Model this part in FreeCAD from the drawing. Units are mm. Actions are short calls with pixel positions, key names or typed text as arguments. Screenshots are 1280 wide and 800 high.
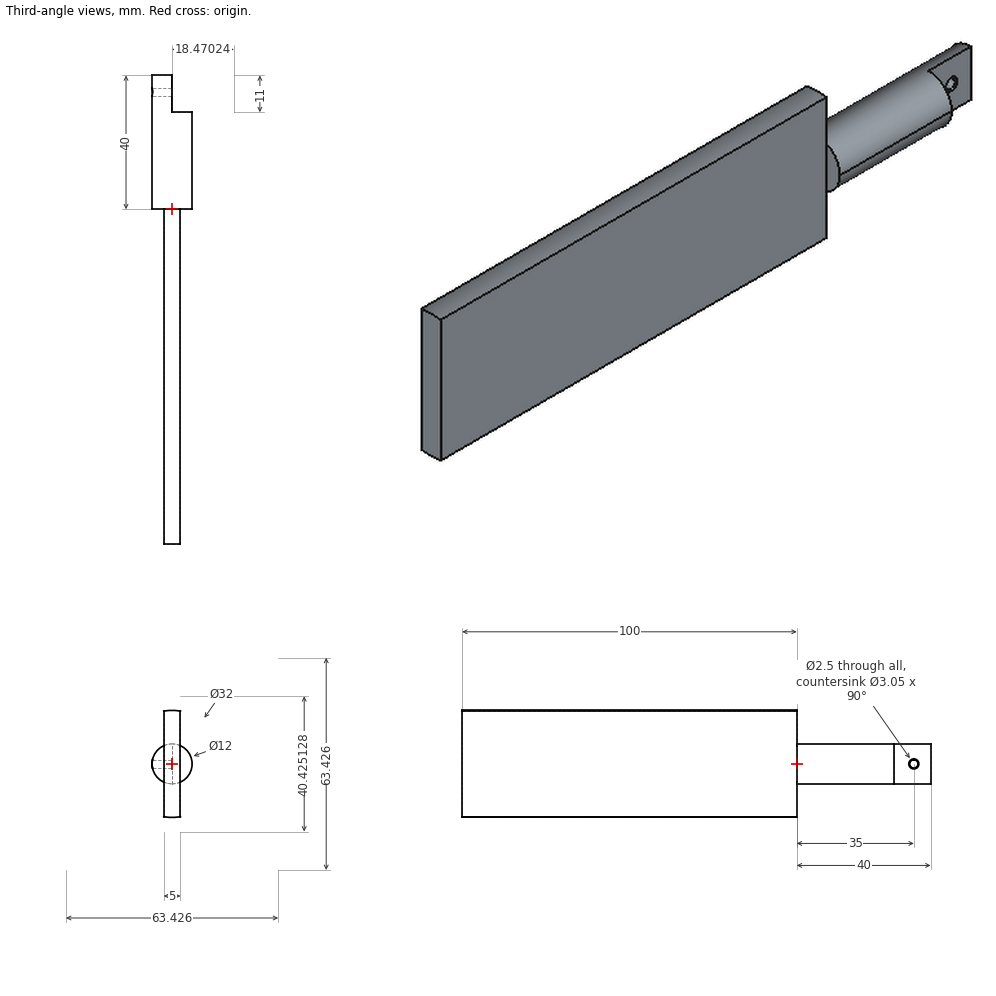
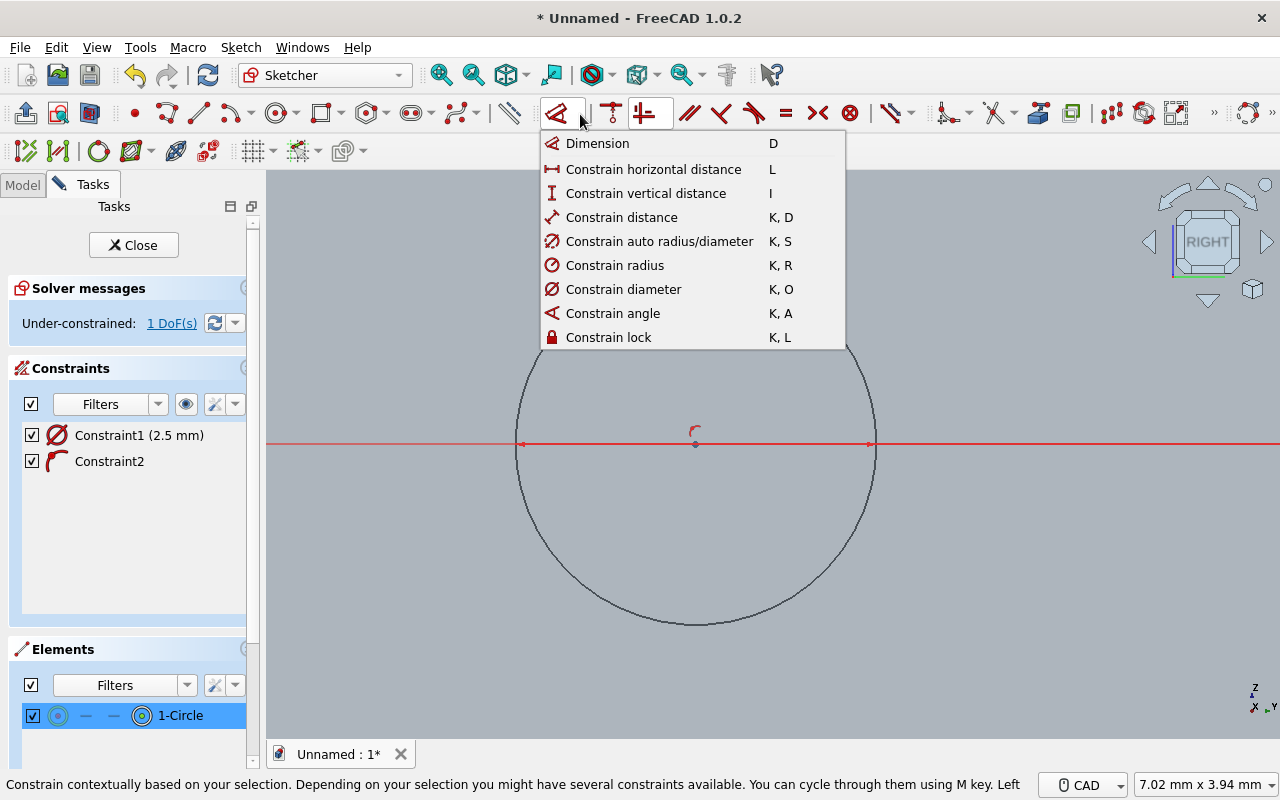
click(693, 169)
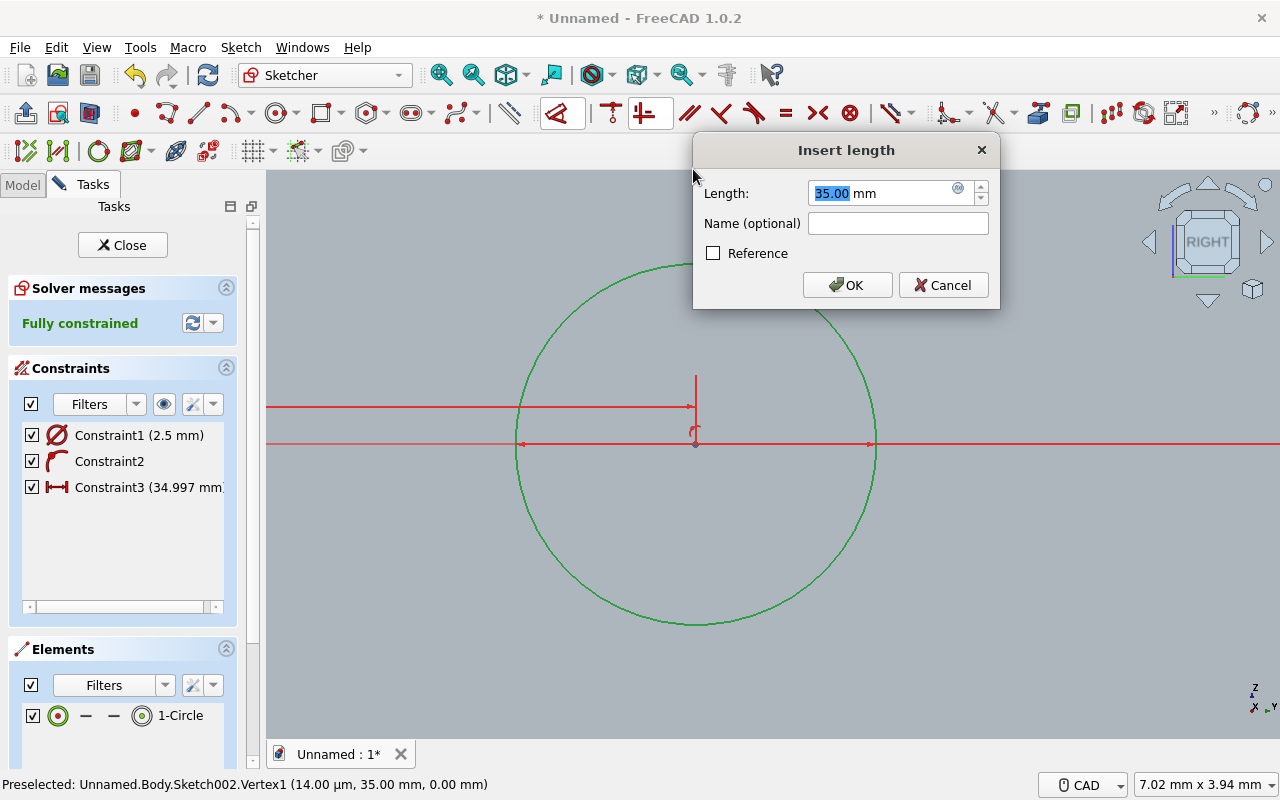
text(35)
key(Return)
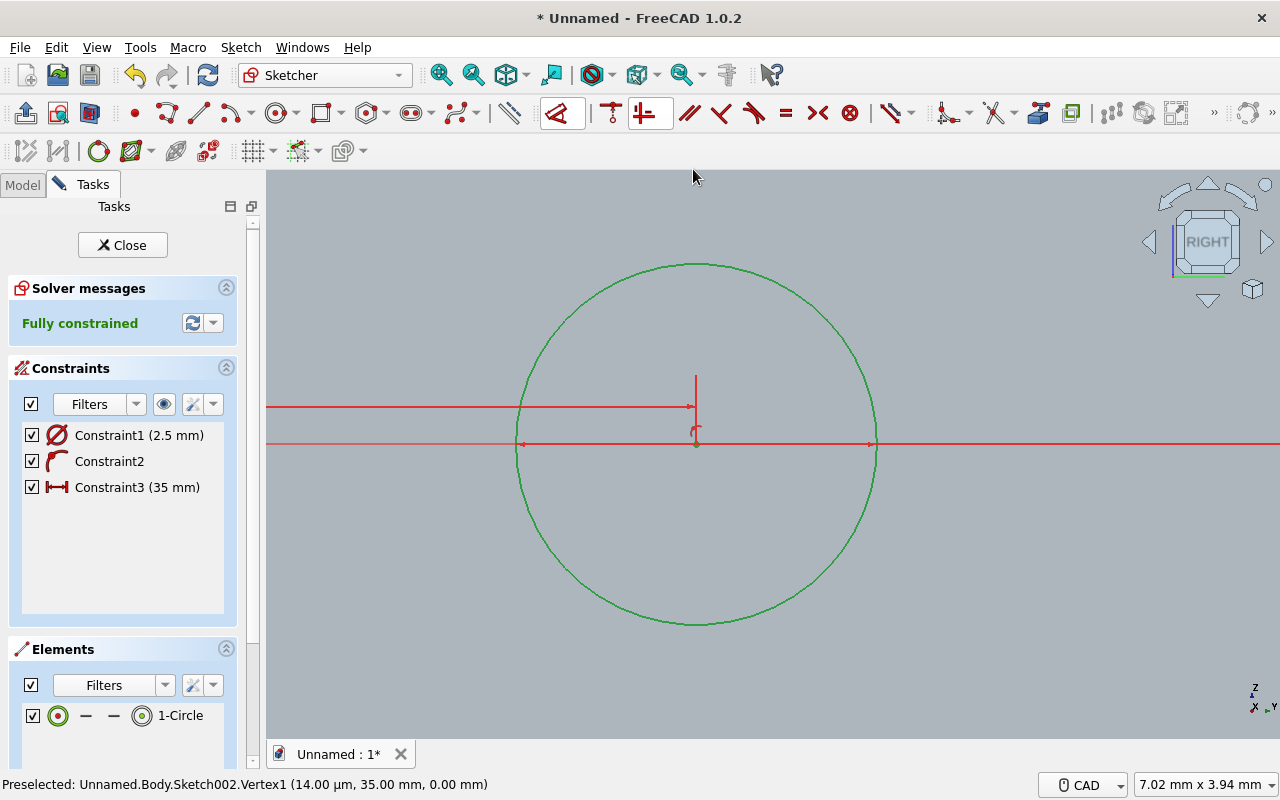
click(123, 245)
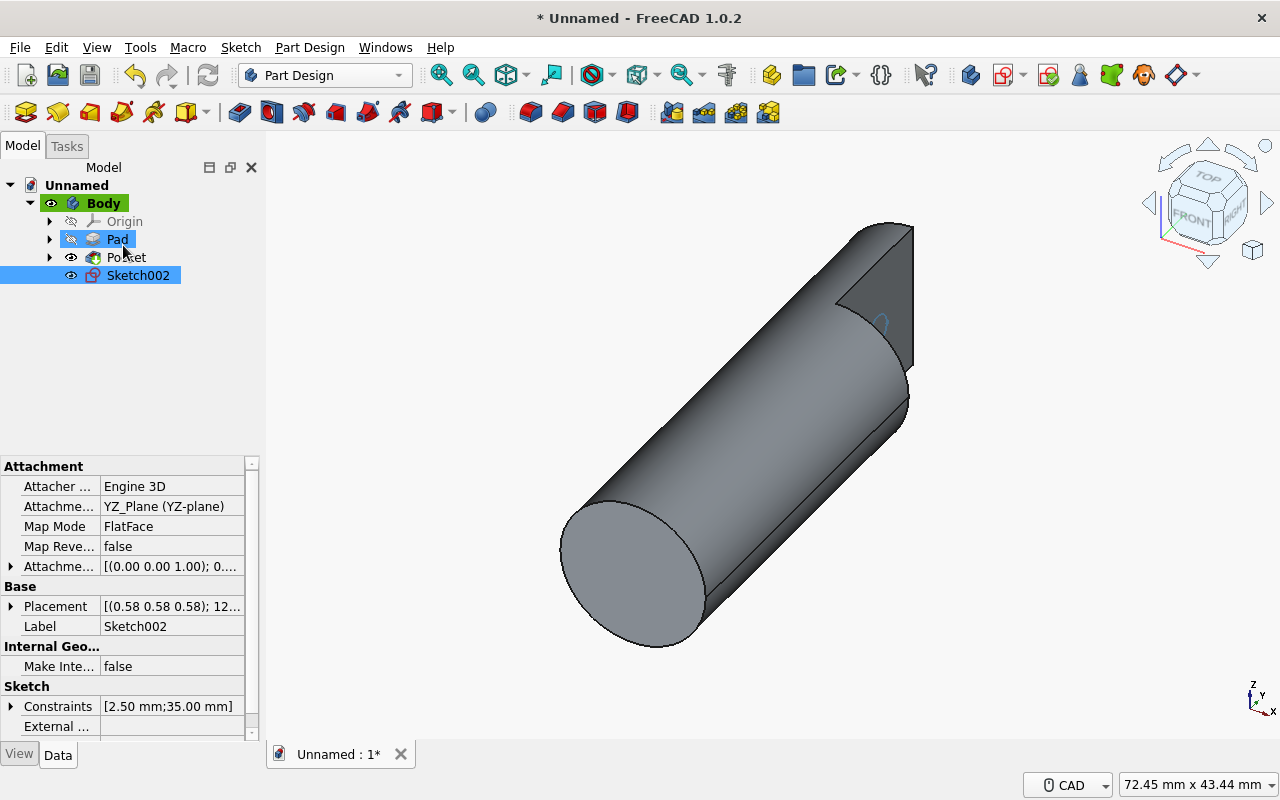
click(272, 112)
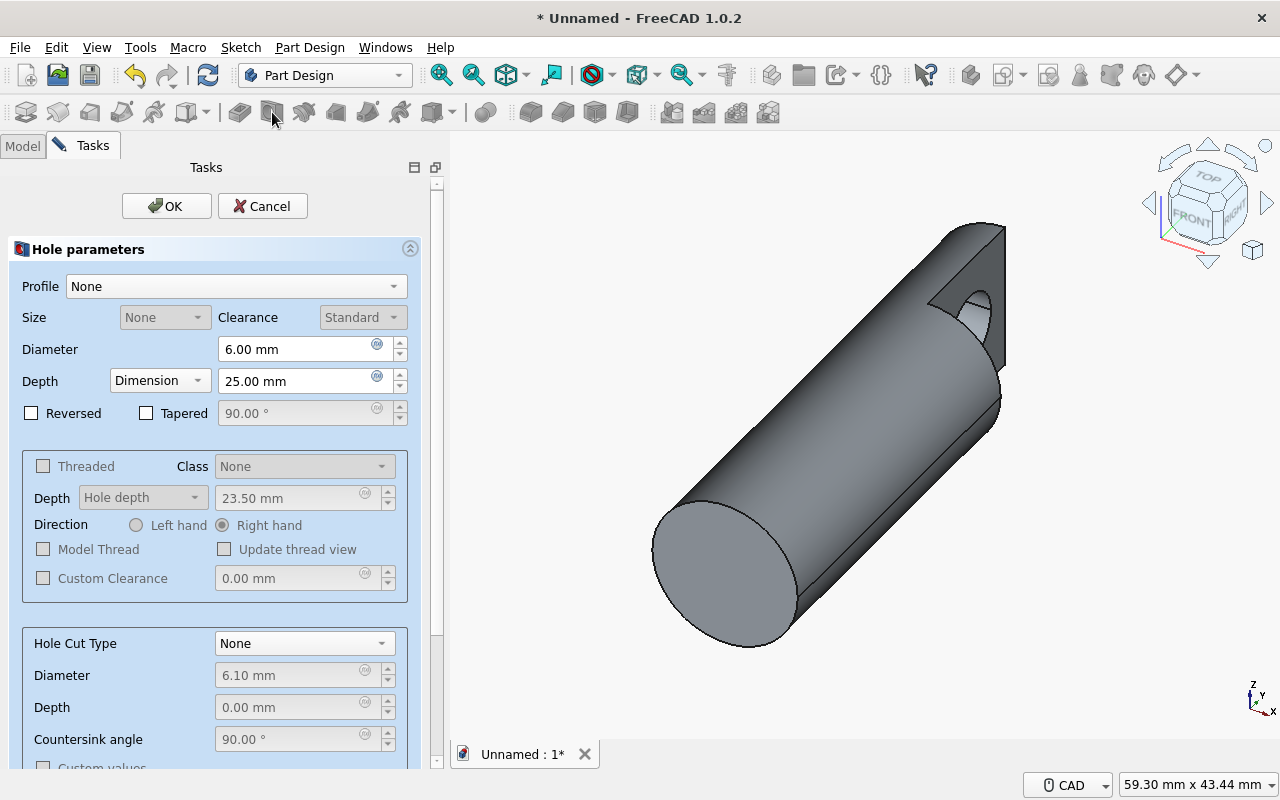
triple_click(305, 349)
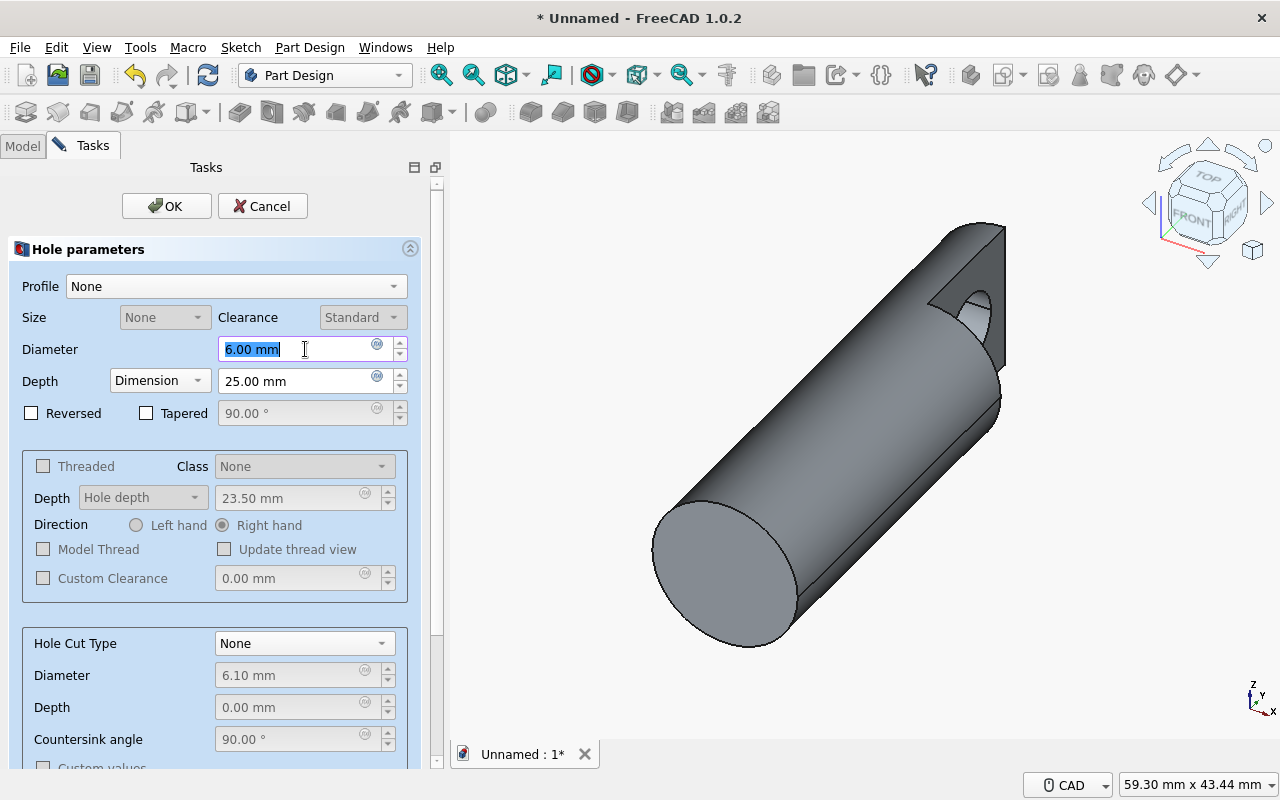
text(2.5)
key(Tab)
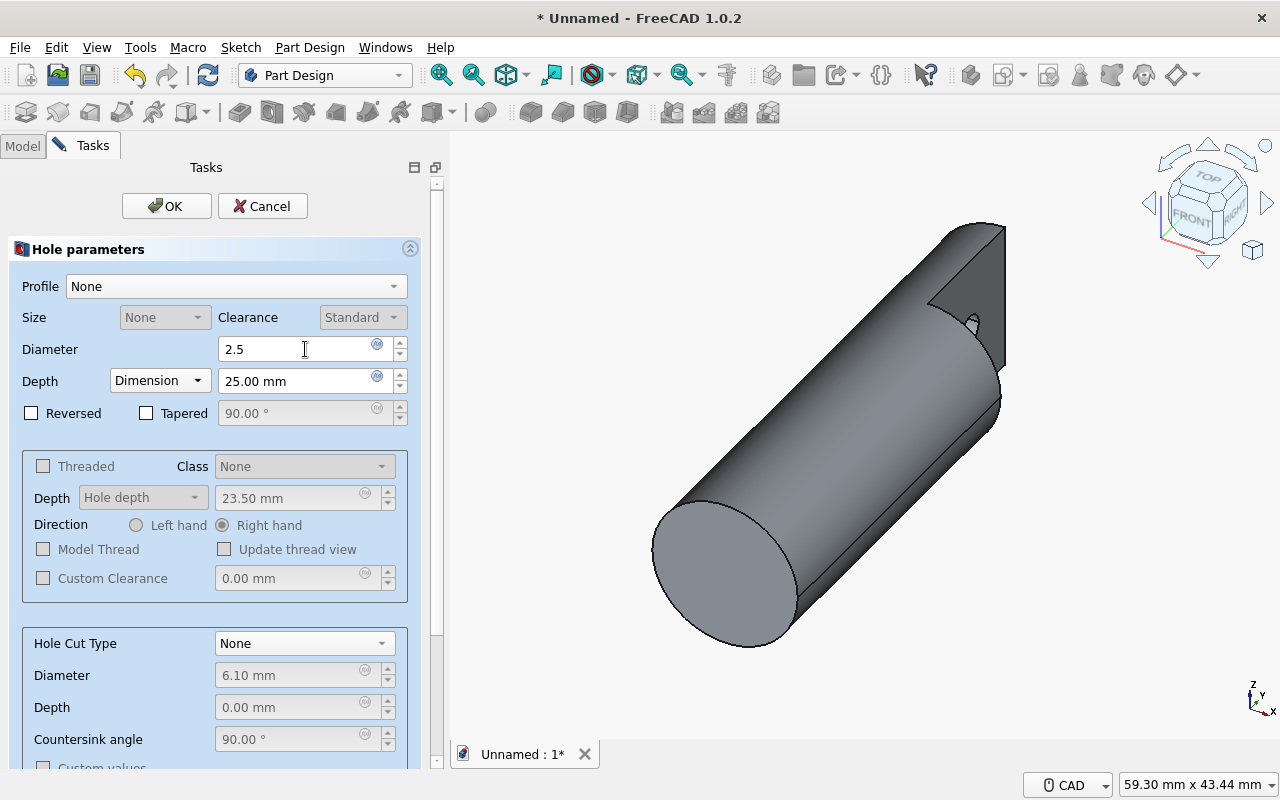
click(161, 380)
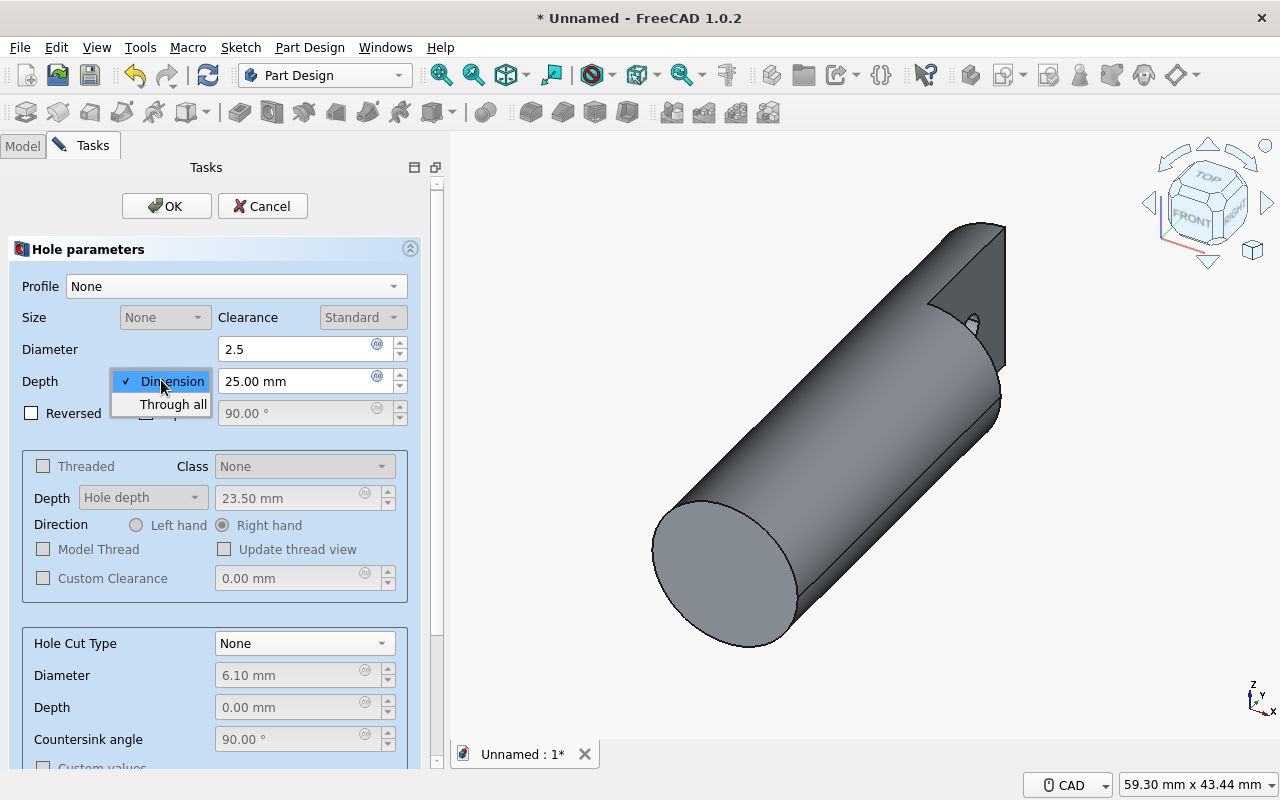
click(160, 404)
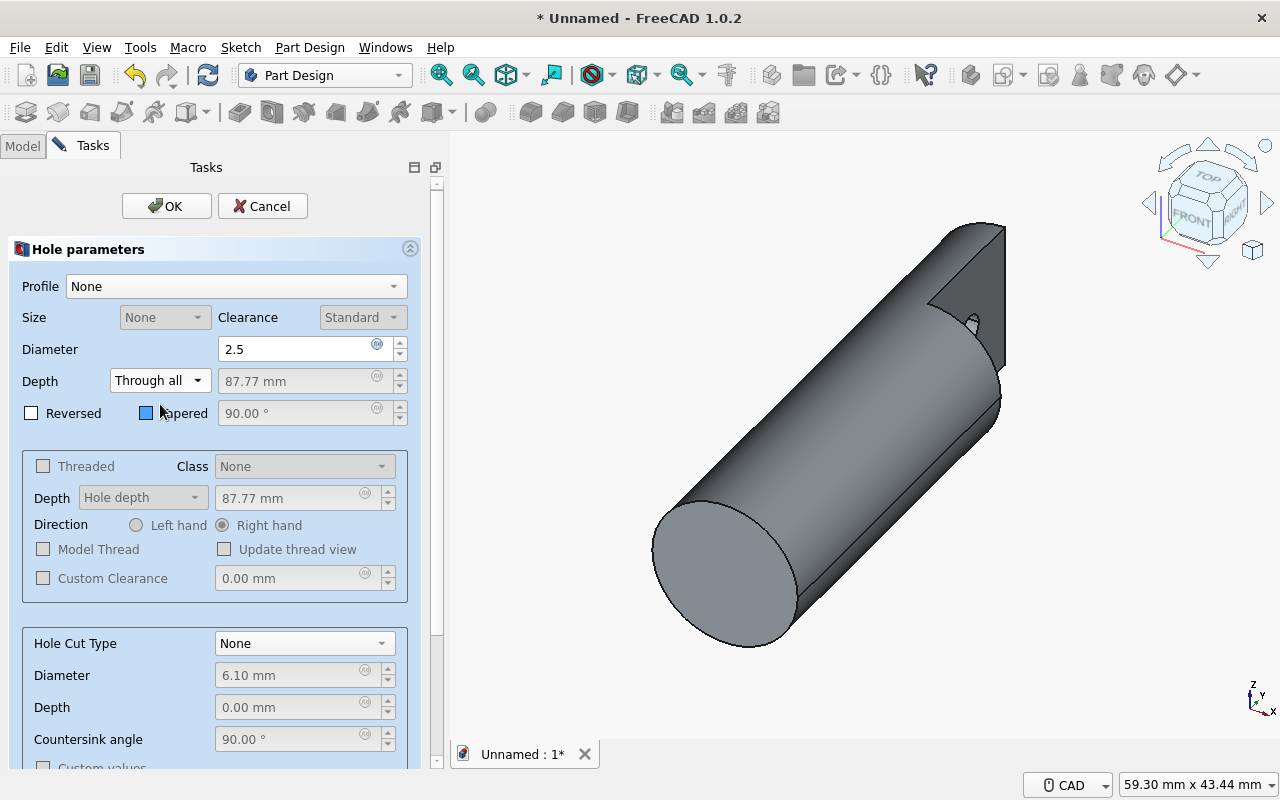
click(306, 644)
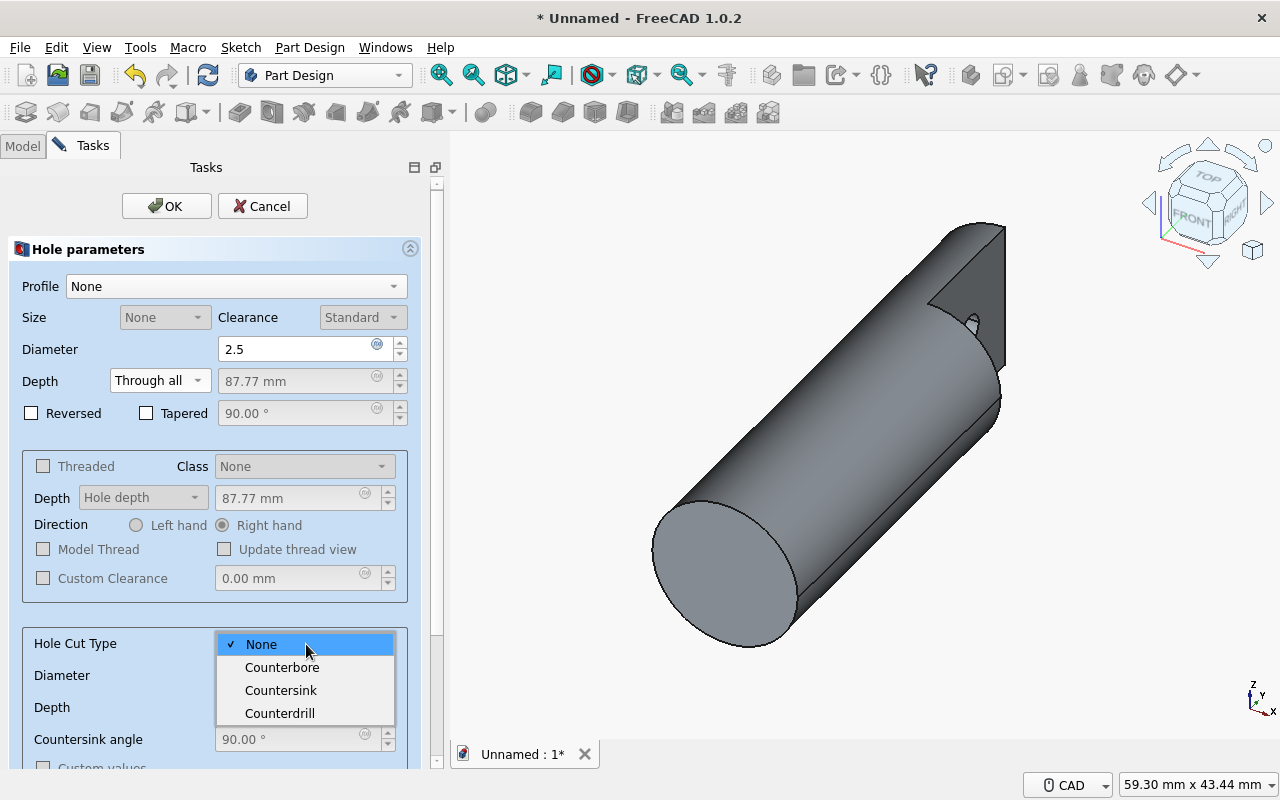
click(304, 690)